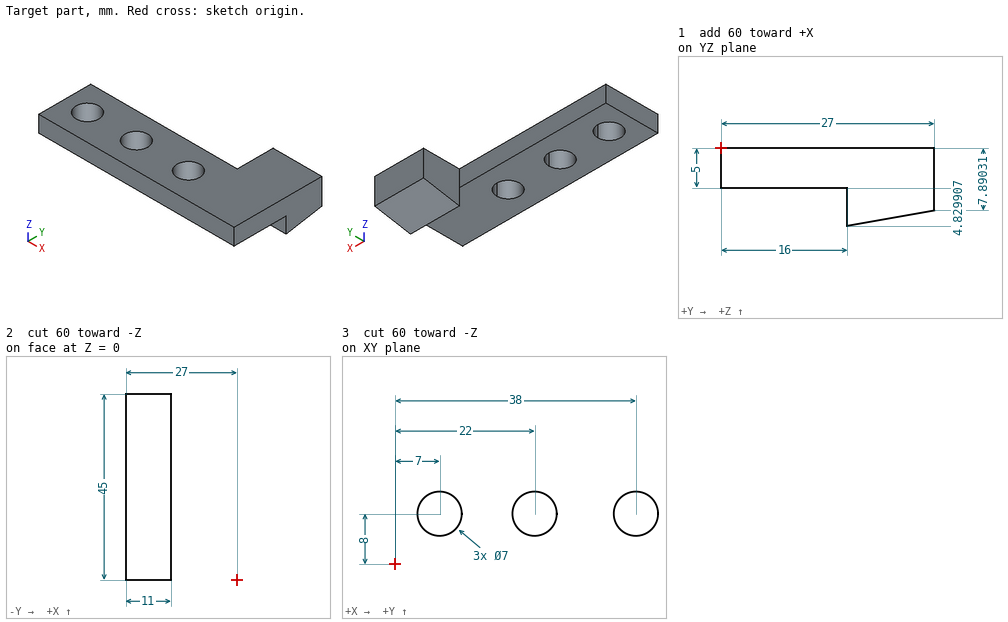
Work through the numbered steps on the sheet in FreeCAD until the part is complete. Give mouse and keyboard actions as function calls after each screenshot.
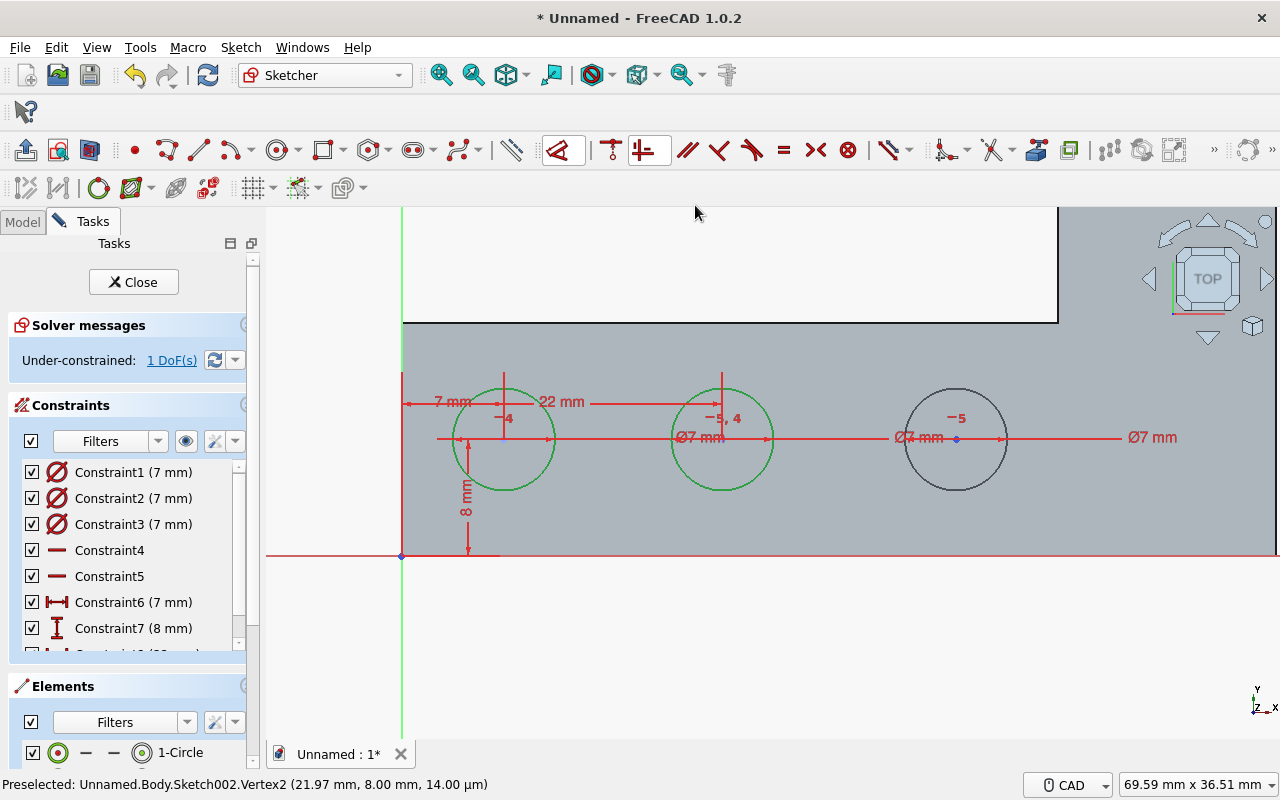
click(956, 439)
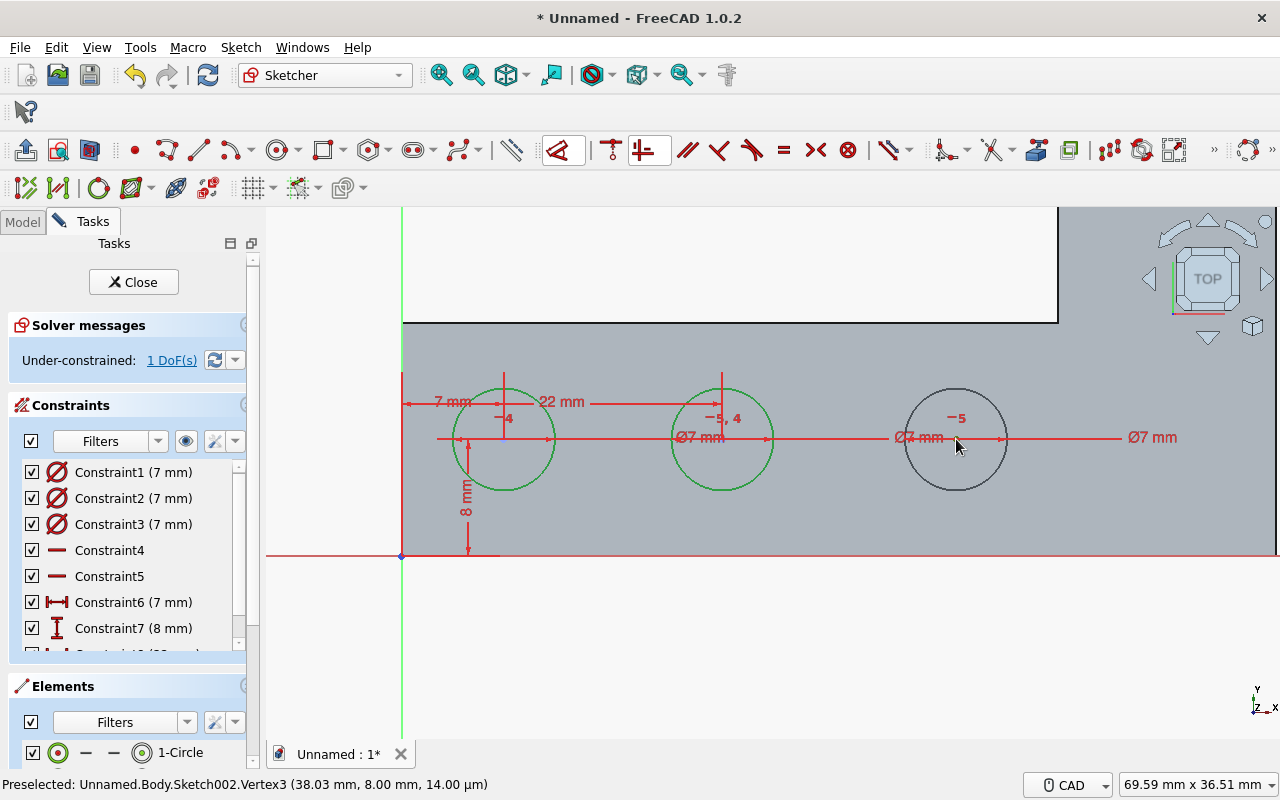
click(580, 150)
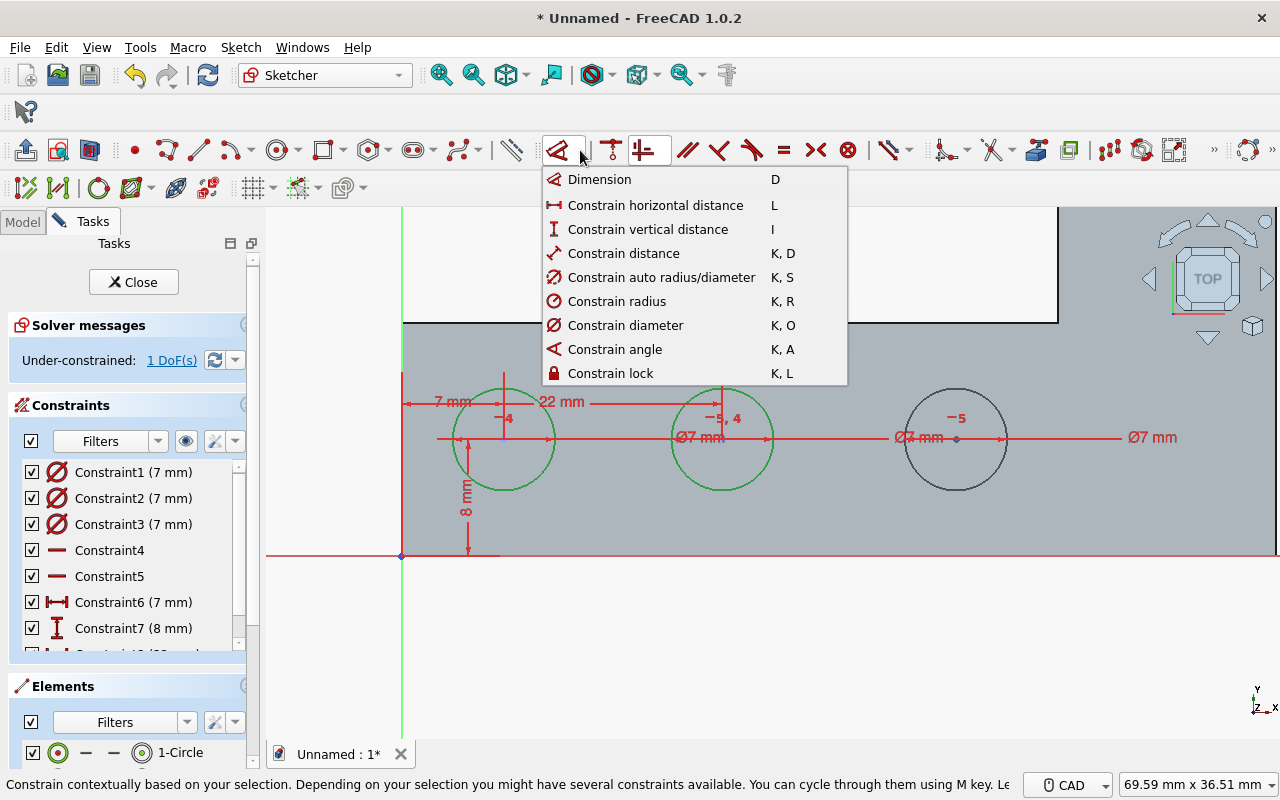
click(695, 205)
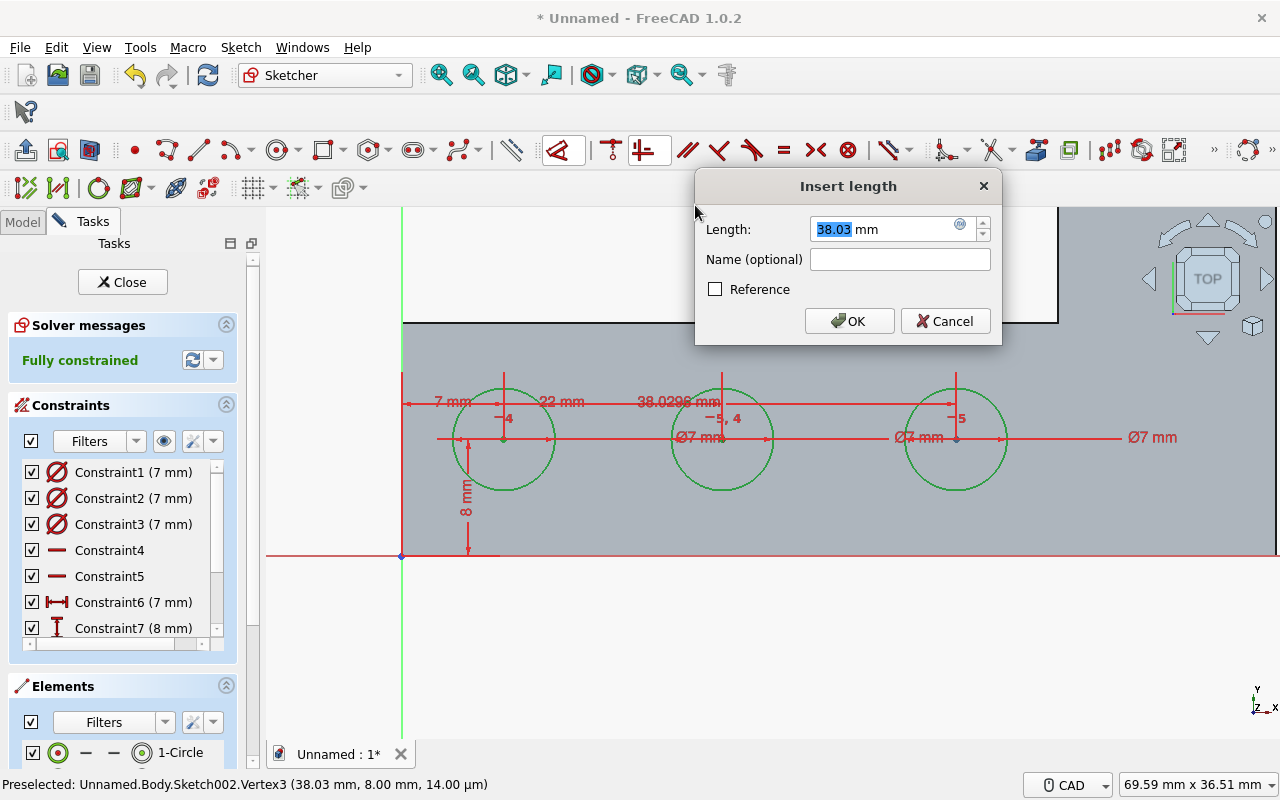
text(38)
key(Return)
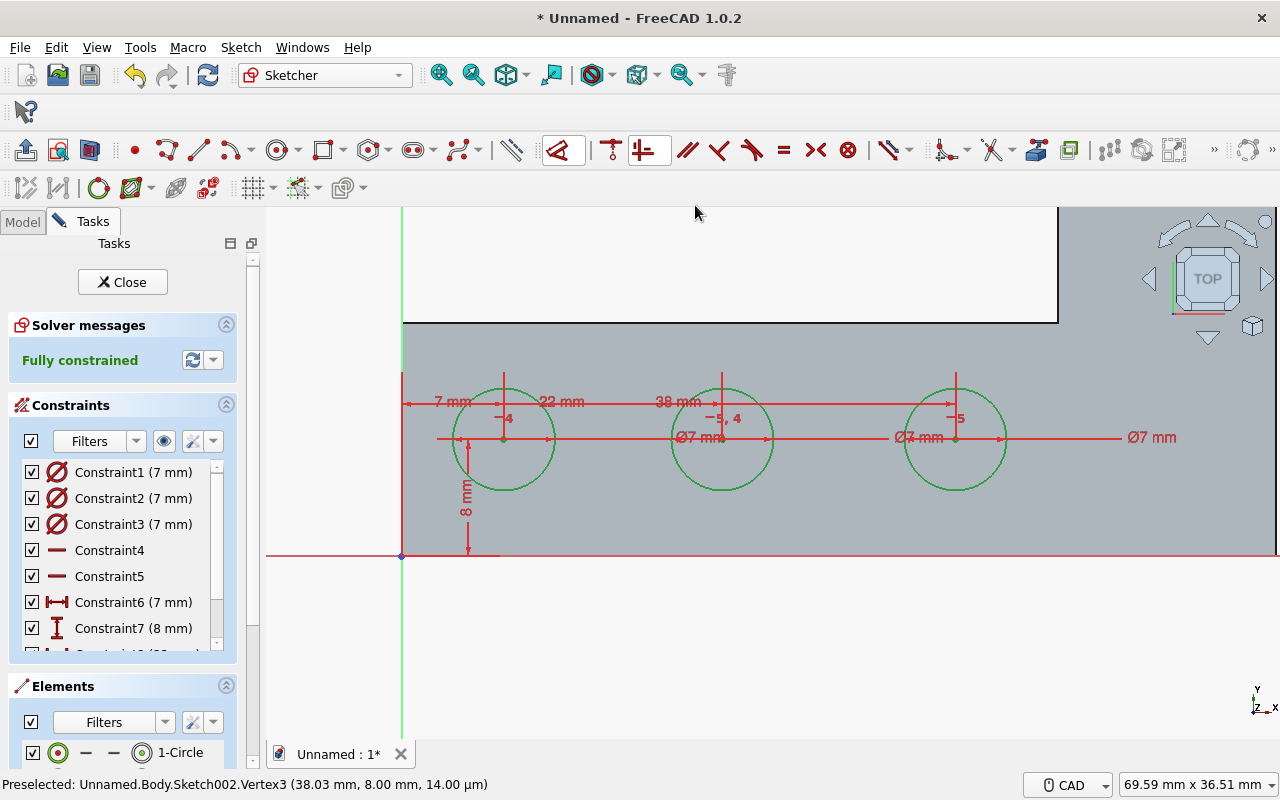
click(123, 282)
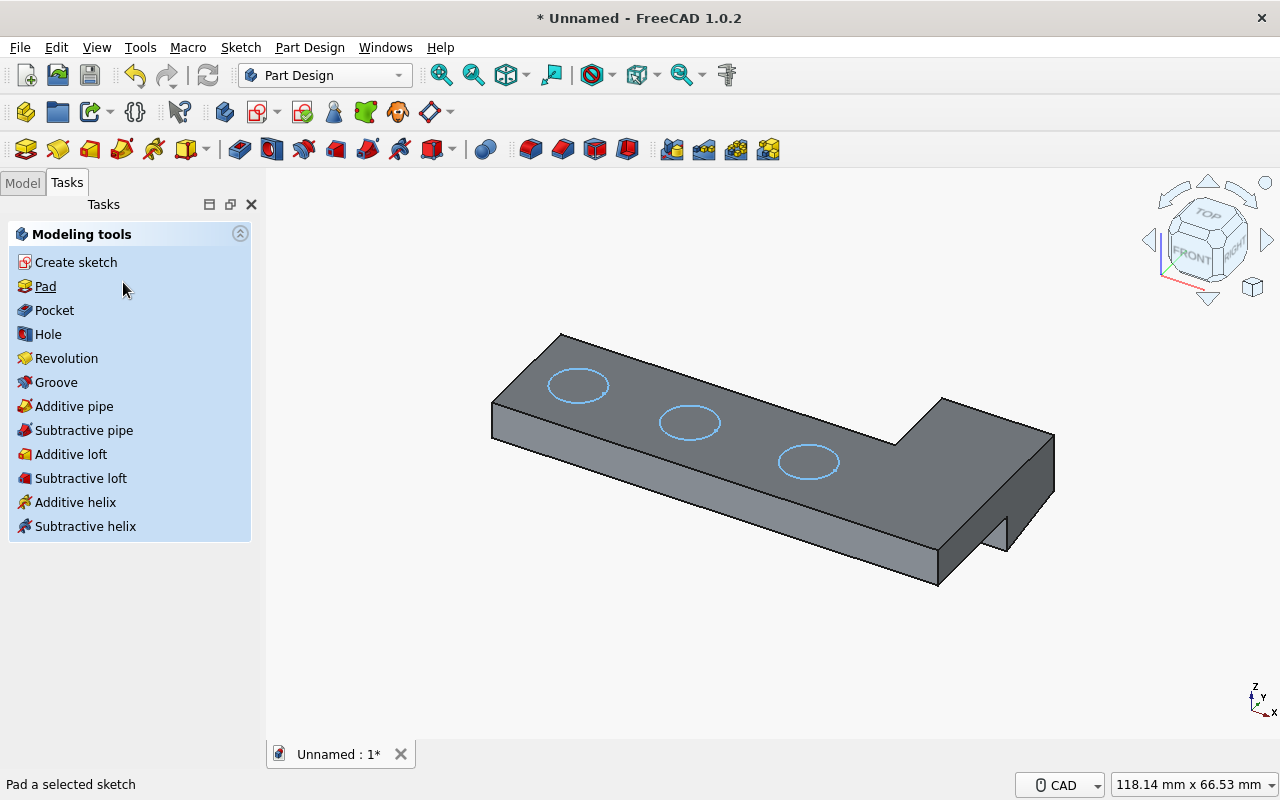
click(240, 150)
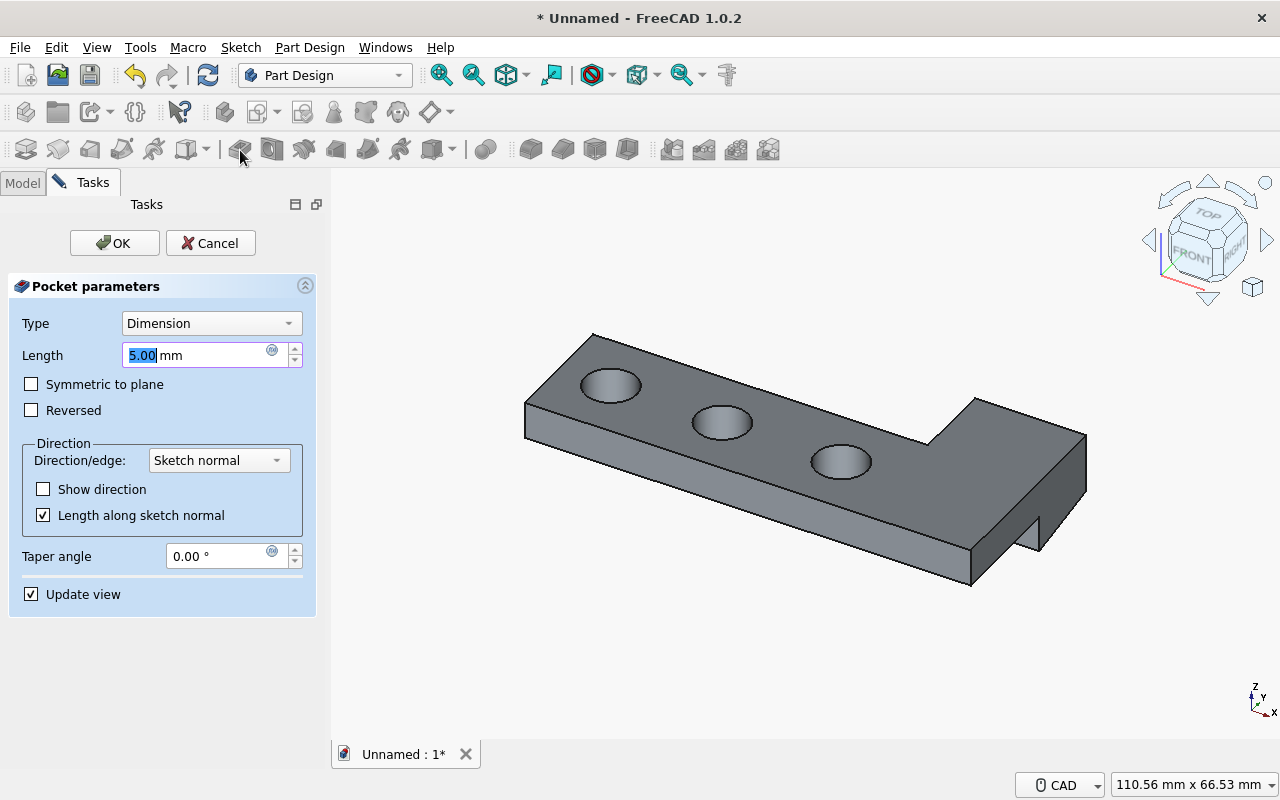
text(60)
key(Tab)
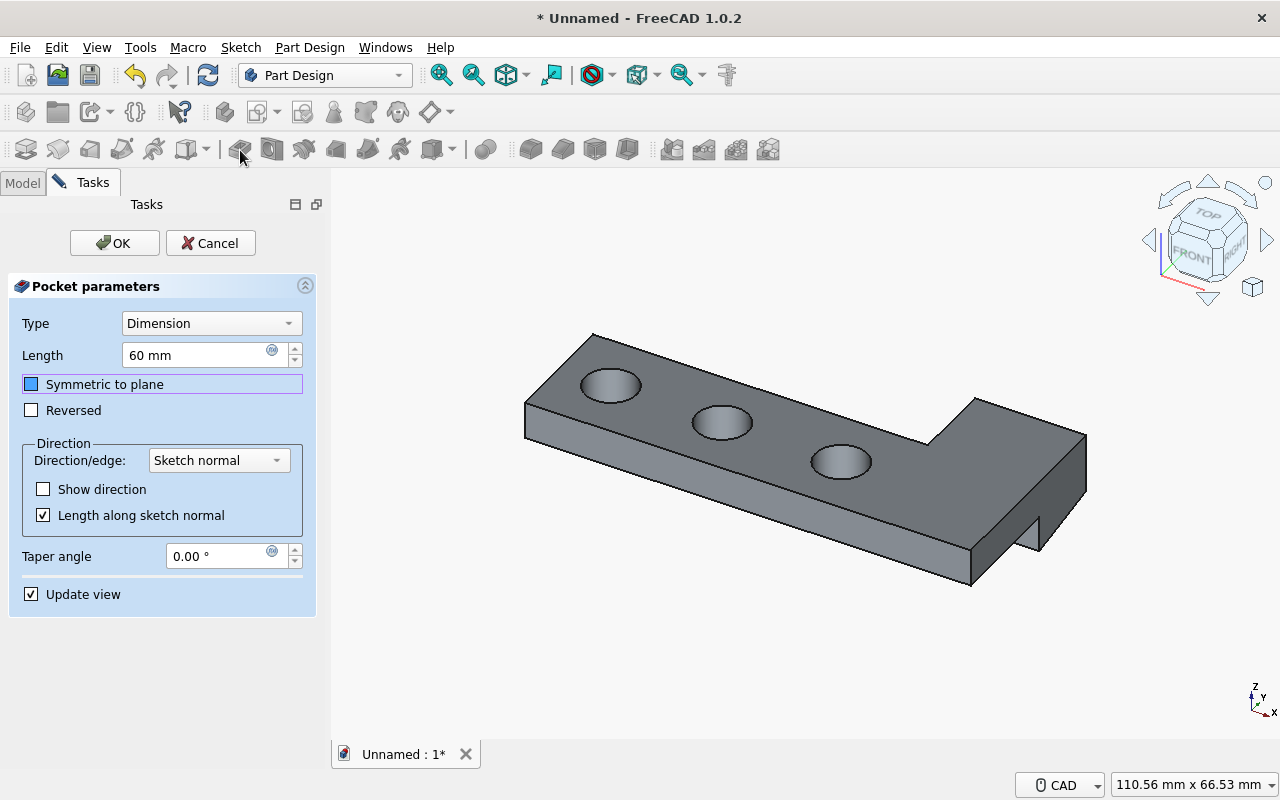
click(115, 243)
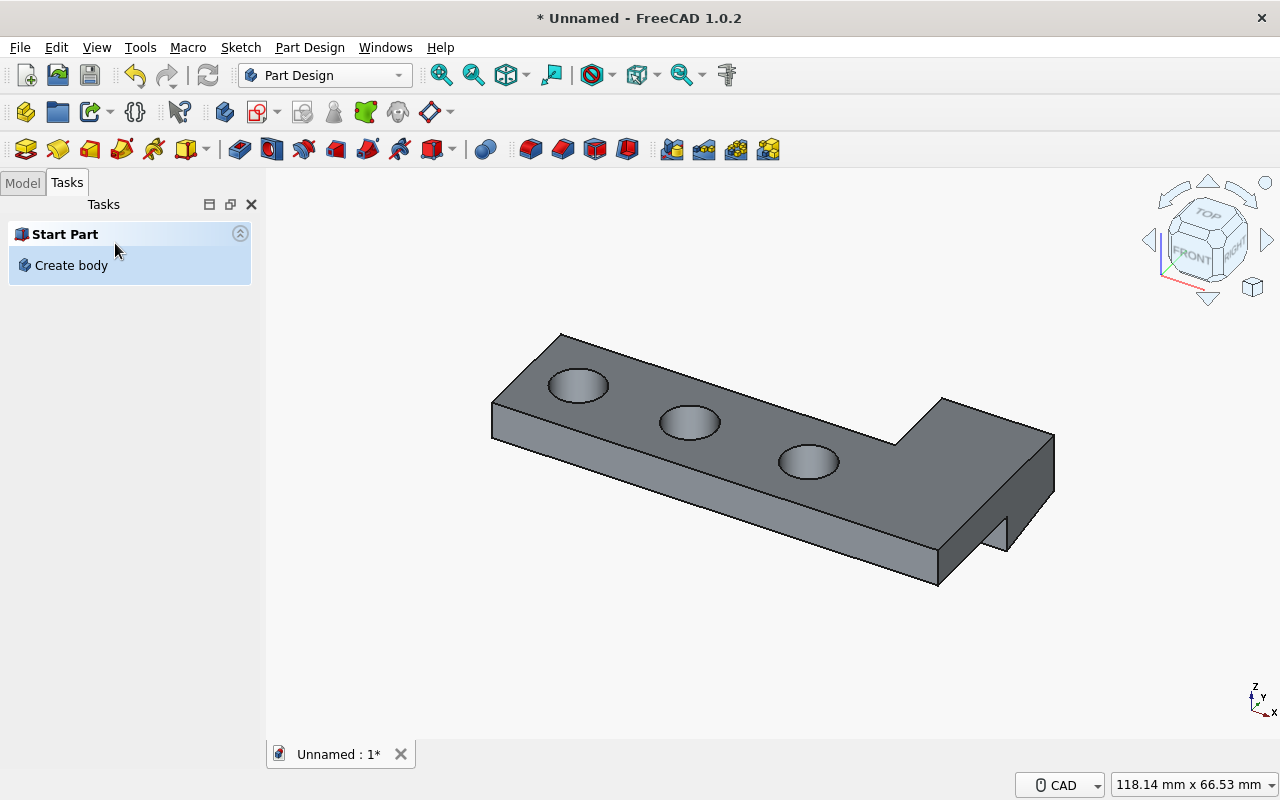
key(0)